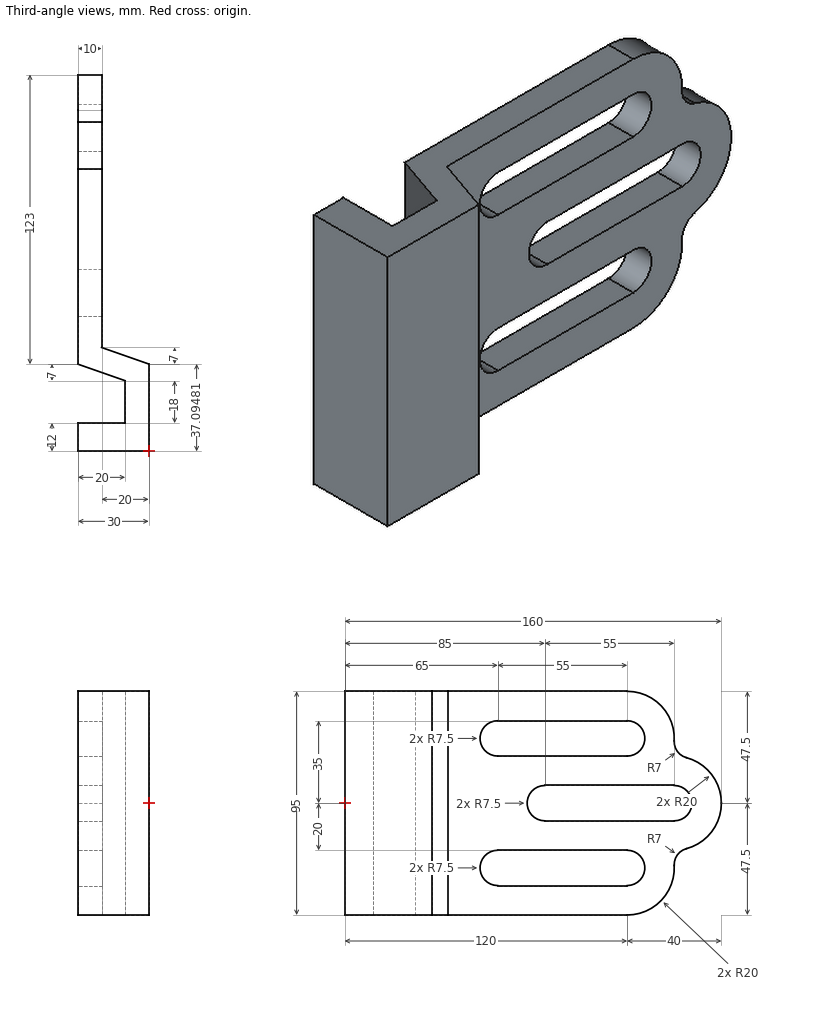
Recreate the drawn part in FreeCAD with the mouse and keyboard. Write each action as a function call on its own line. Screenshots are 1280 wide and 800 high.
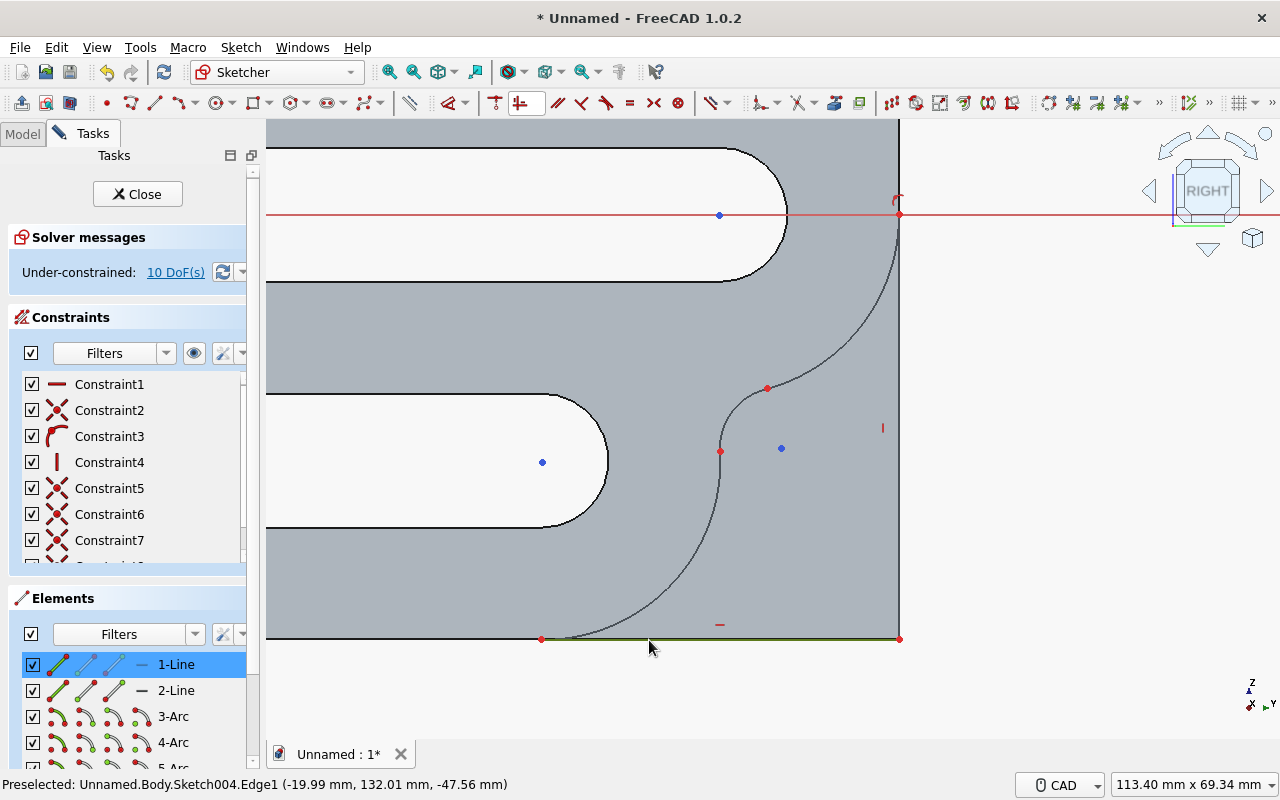
click(626, 619)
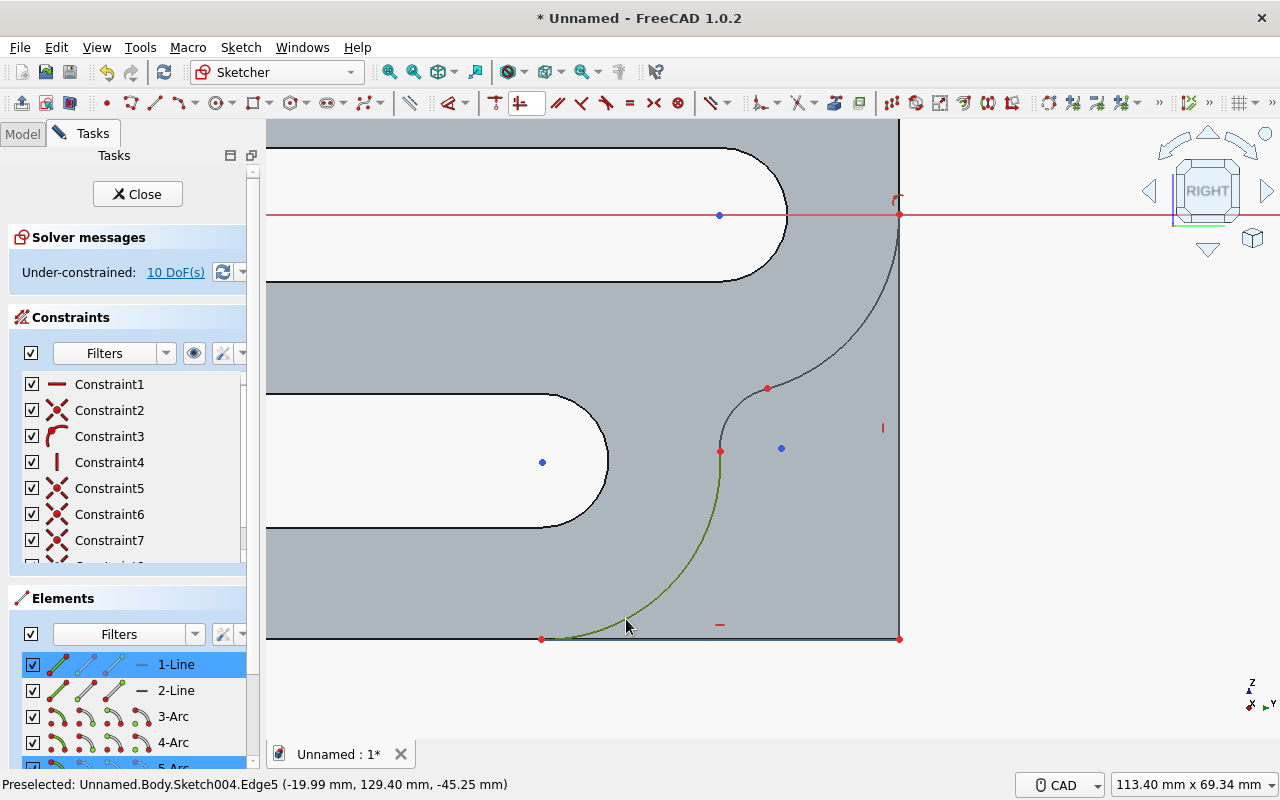
key(t)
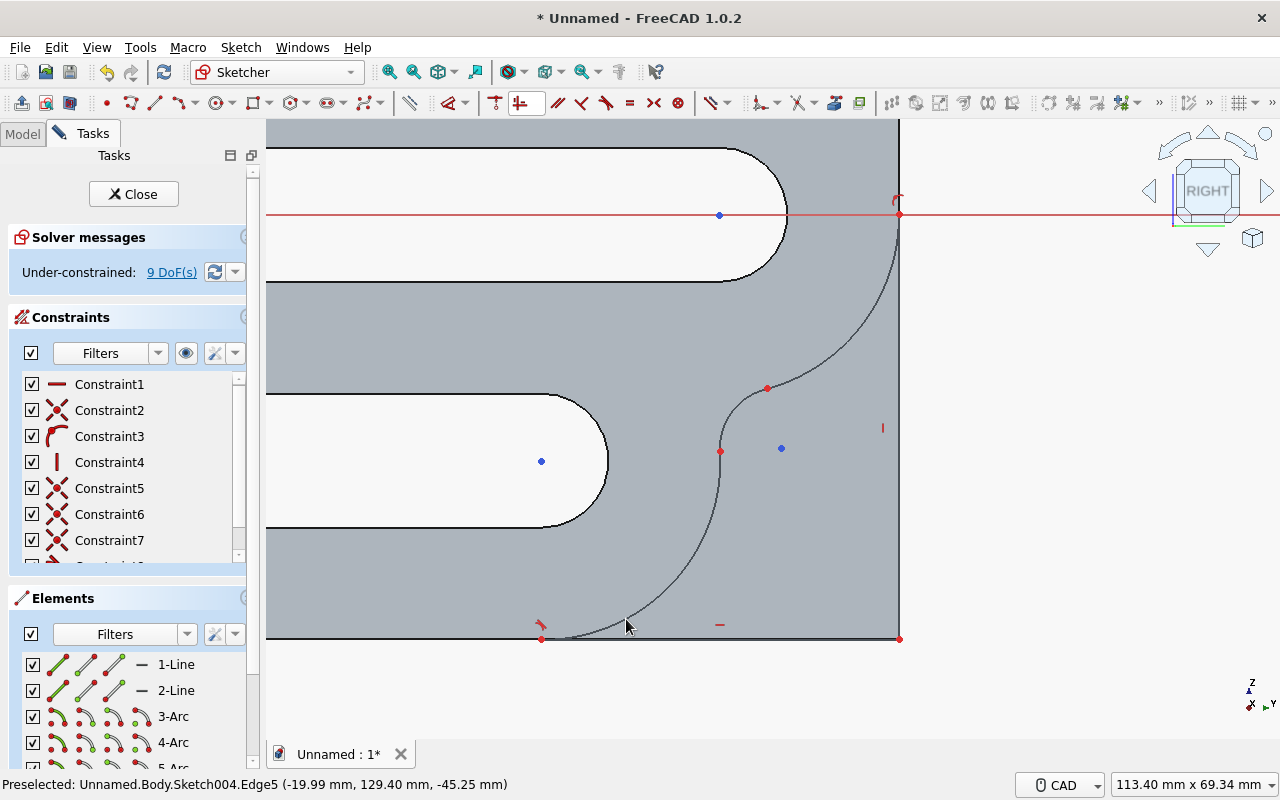
click(899, 512)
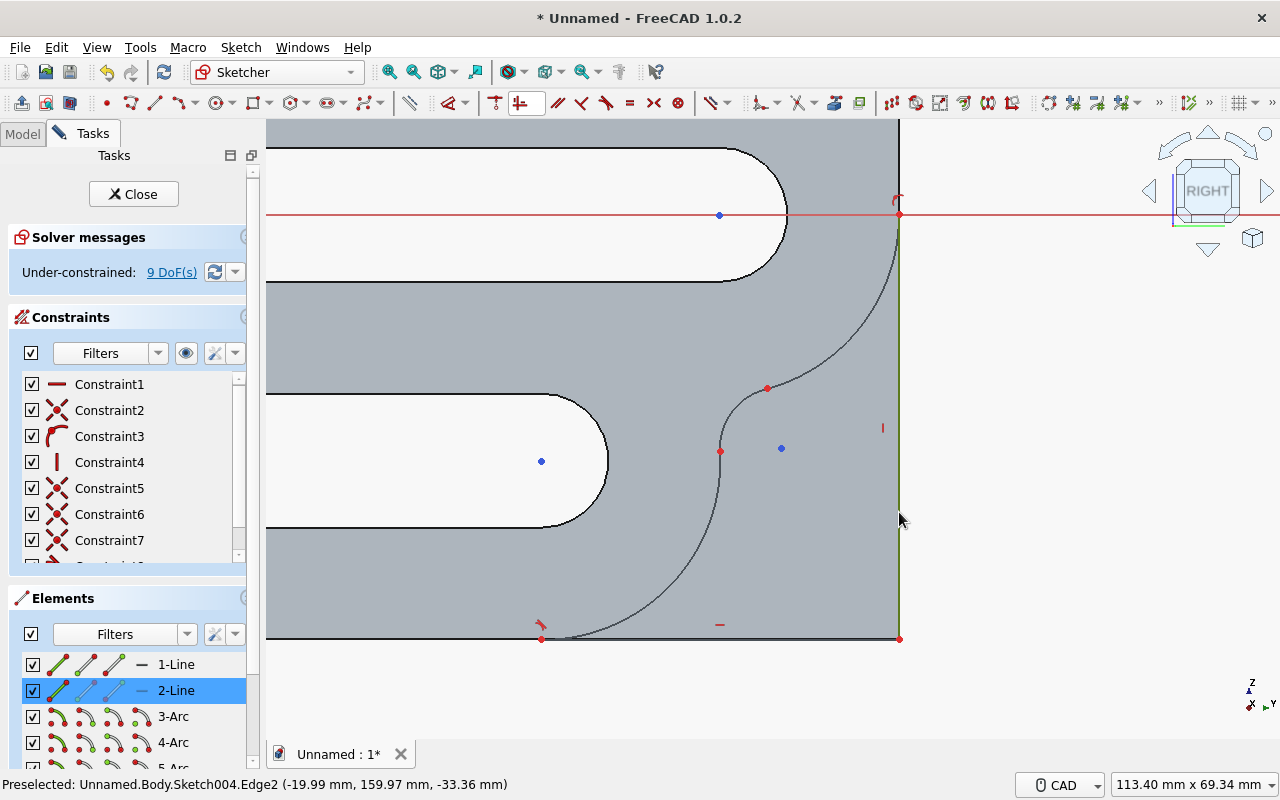
click(830, 358)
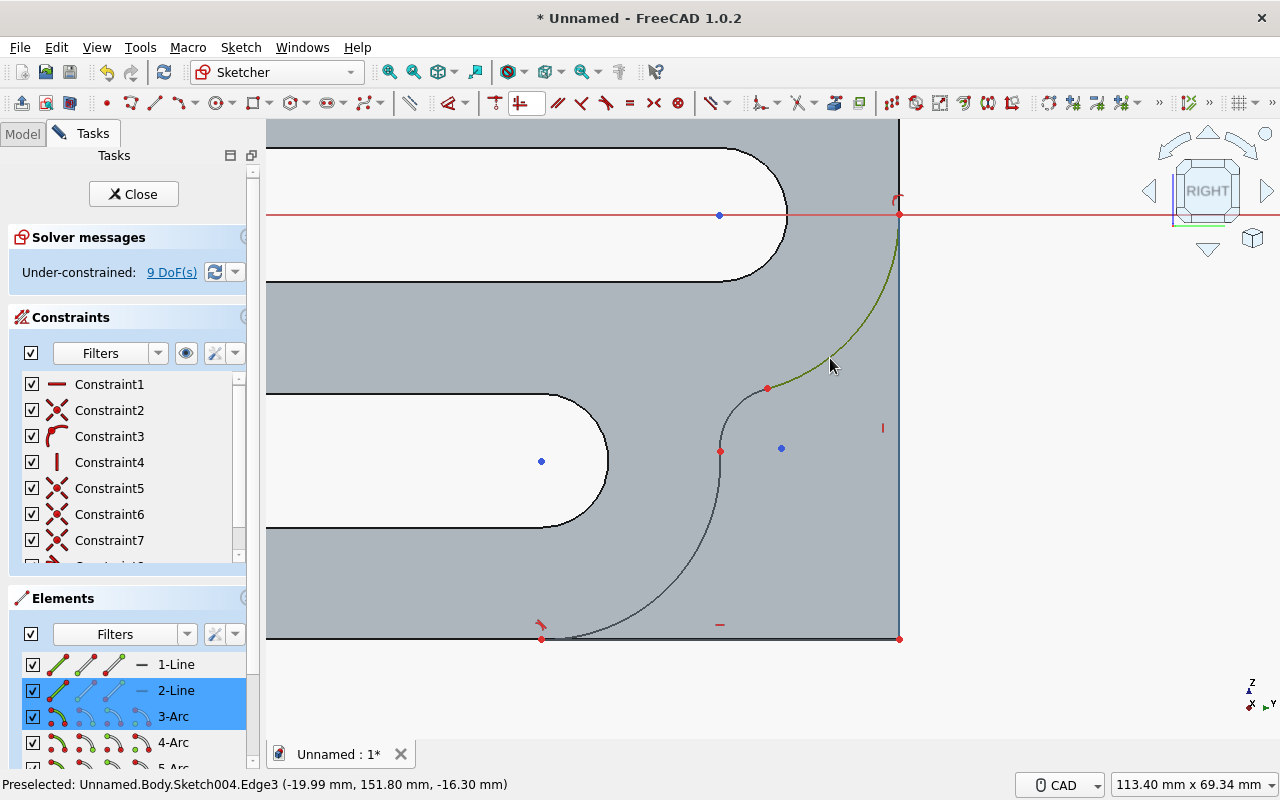
click(606, 104)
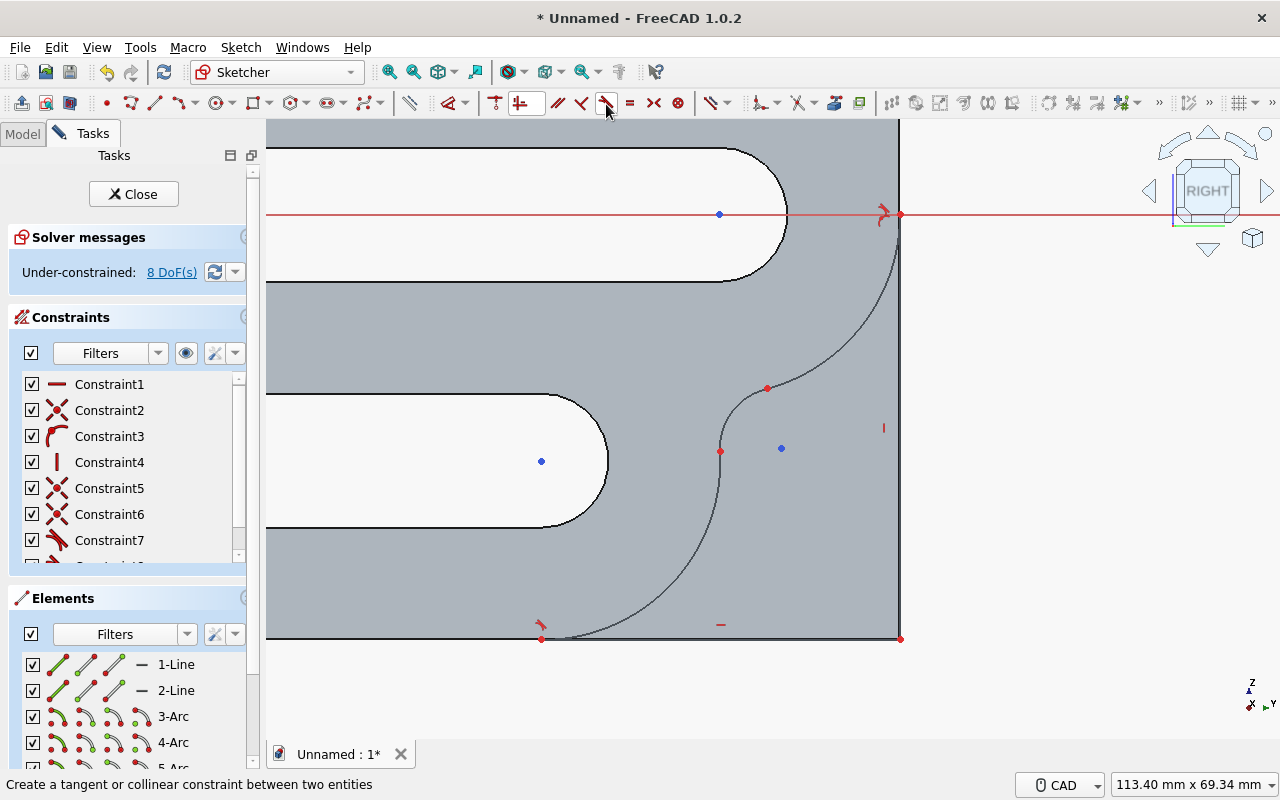
click(830, 358)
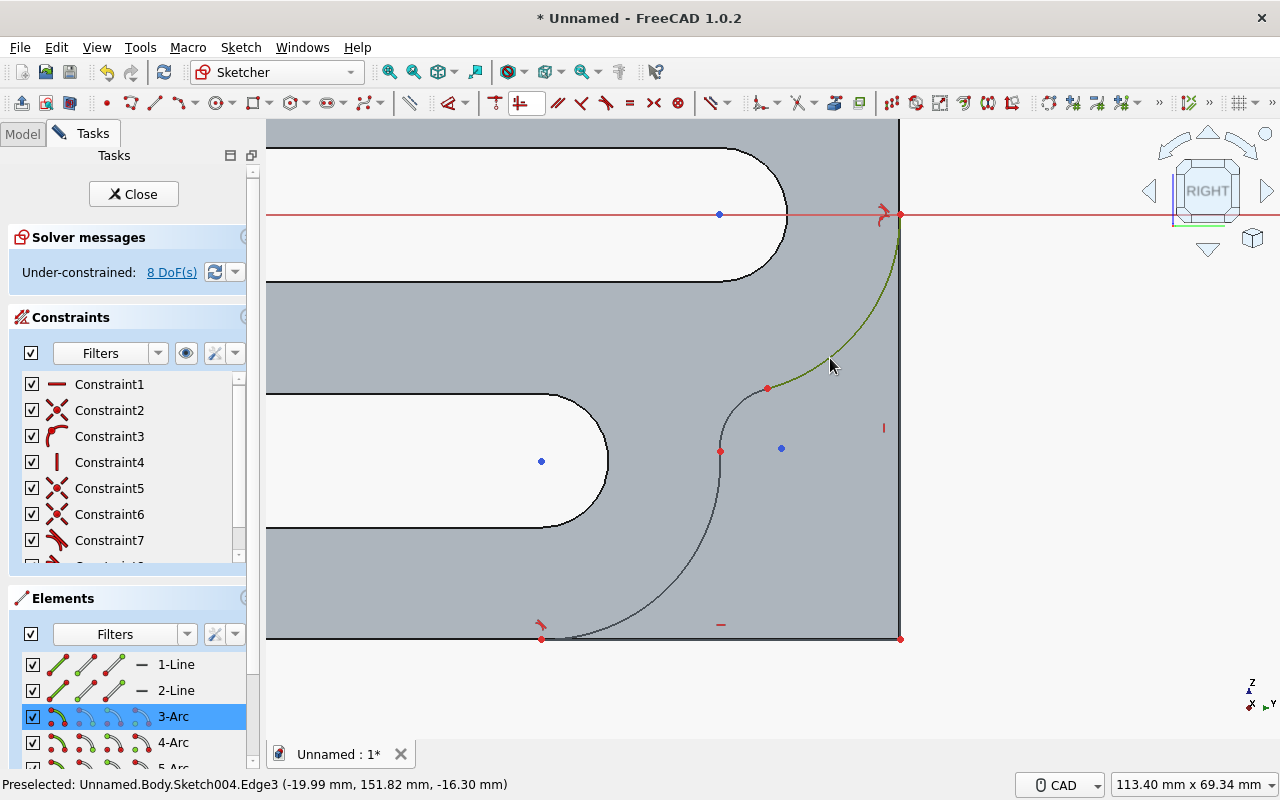
click(744, 400)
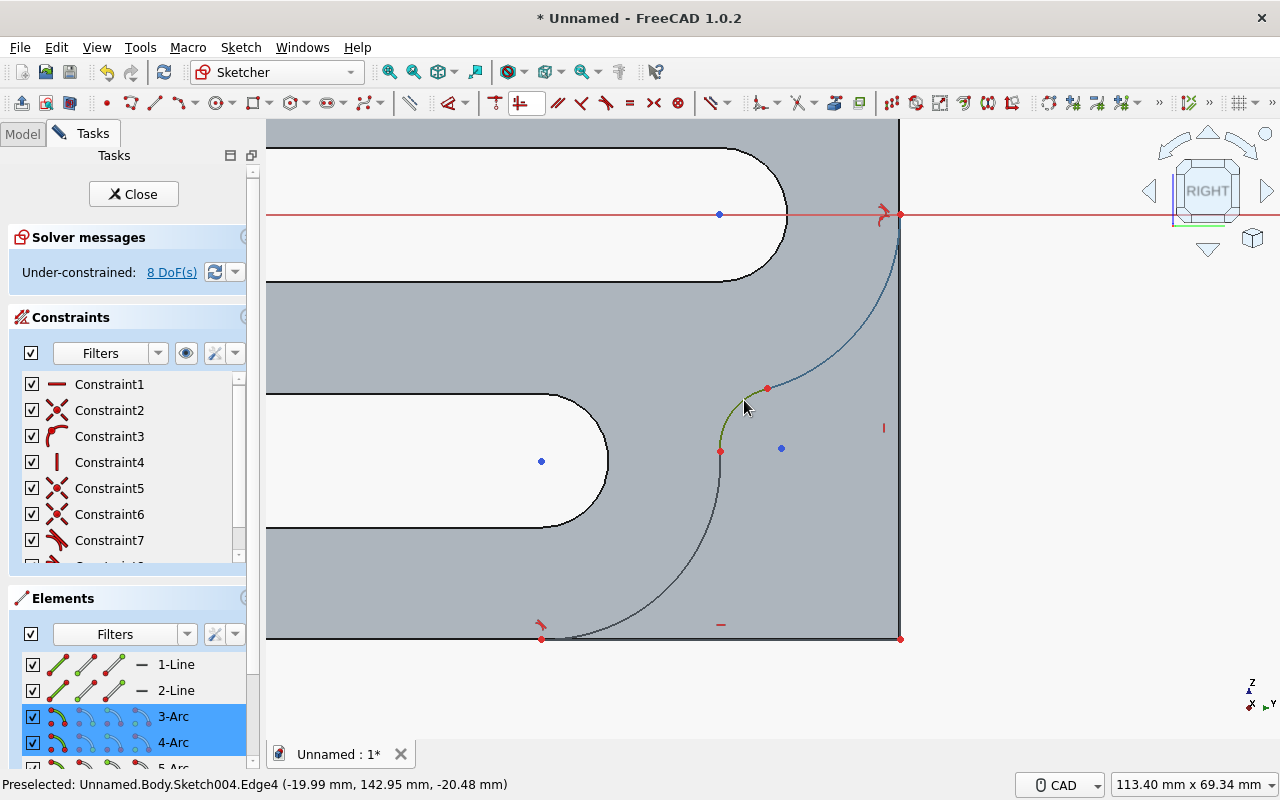
click(606, 104)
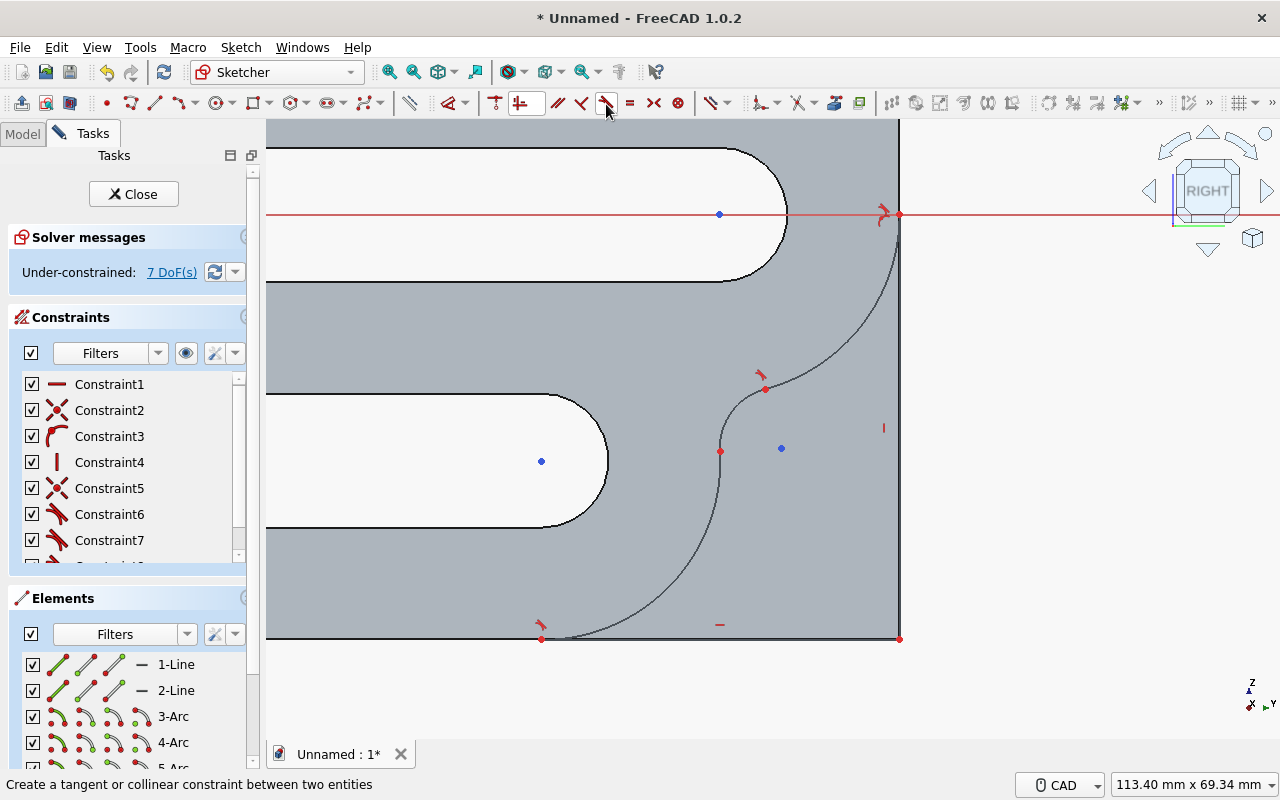
click(743, 400)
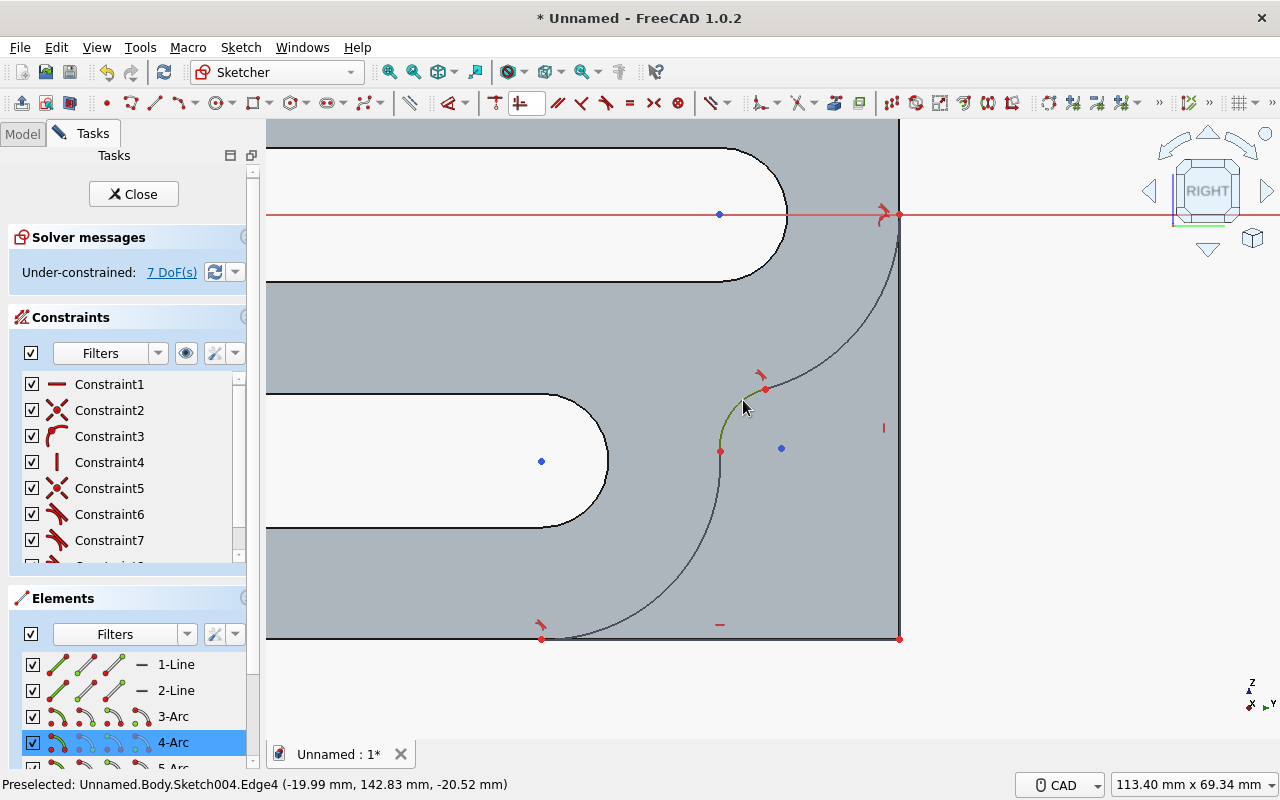
click(626, 619)